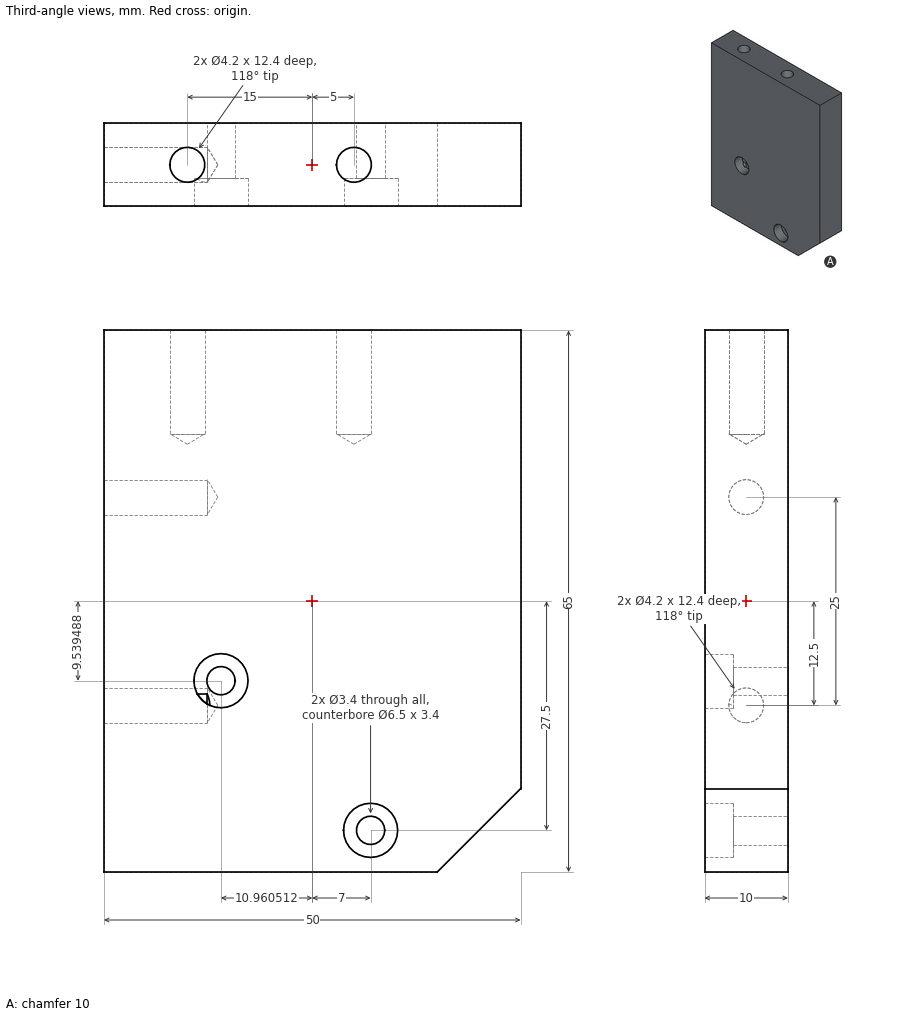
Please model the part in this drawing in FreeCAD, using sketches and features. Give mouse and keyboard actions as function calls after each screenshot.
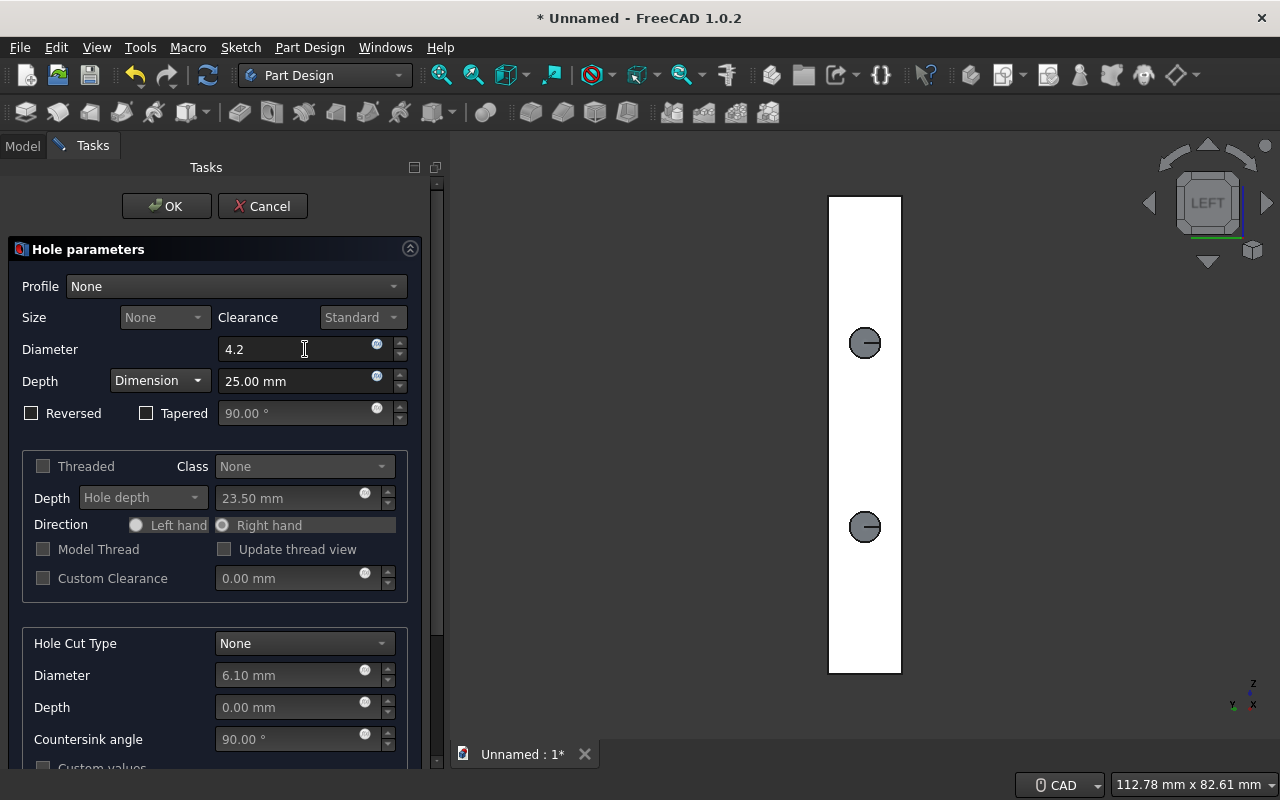
triple_click(305, 381)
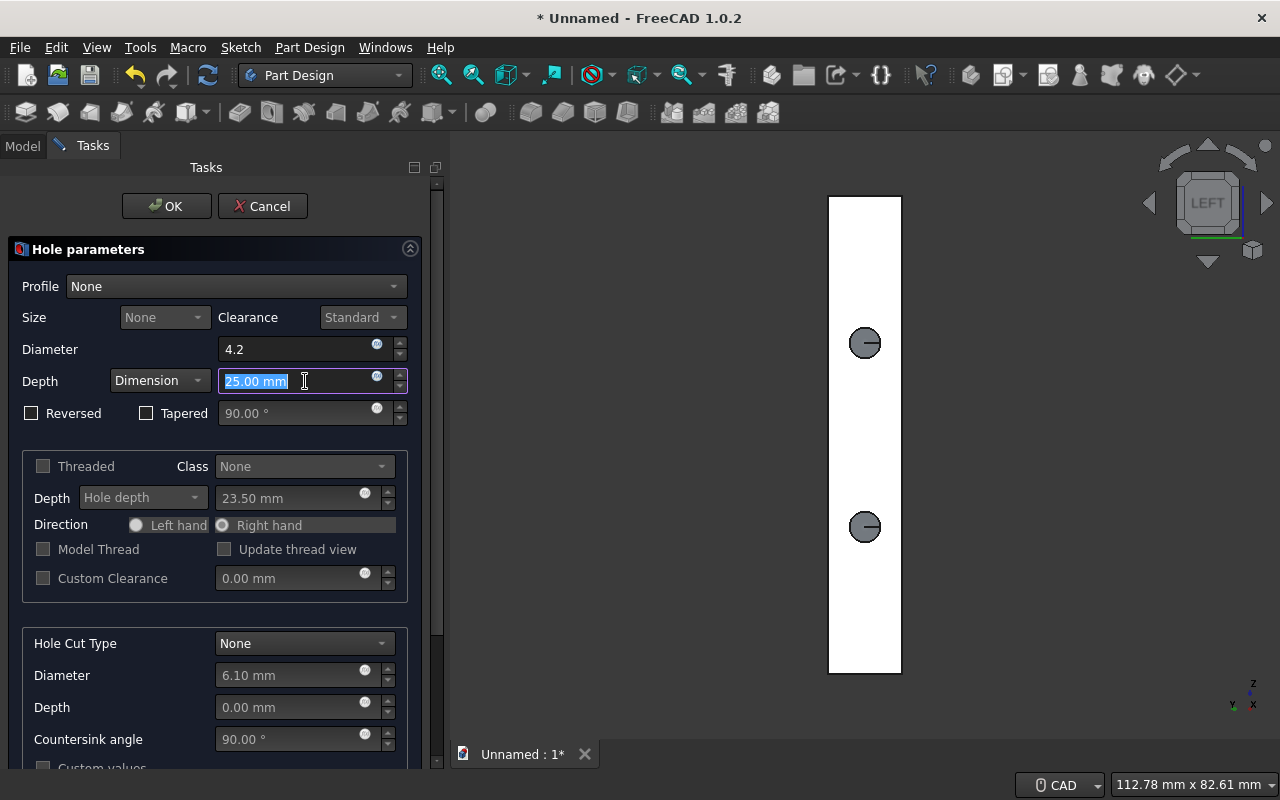
text(12.4)
key(Tab)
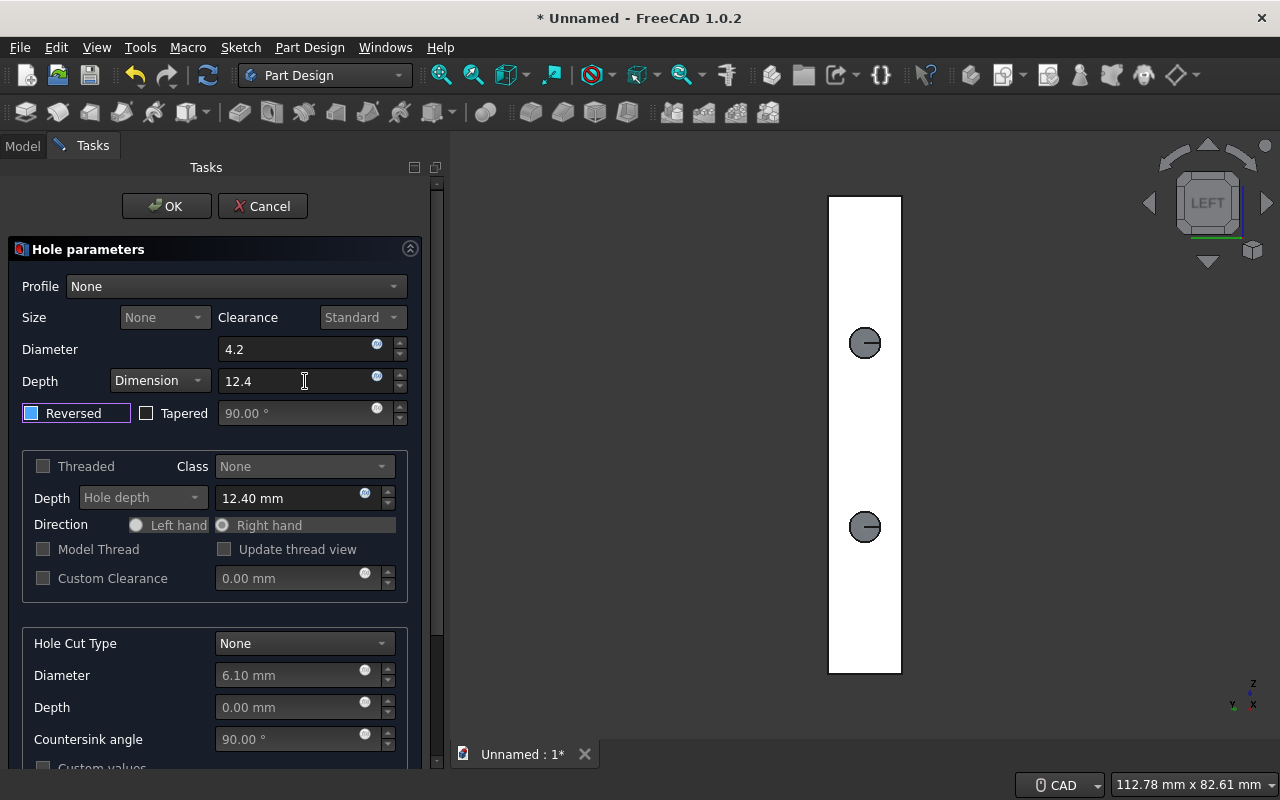
click(167, 206)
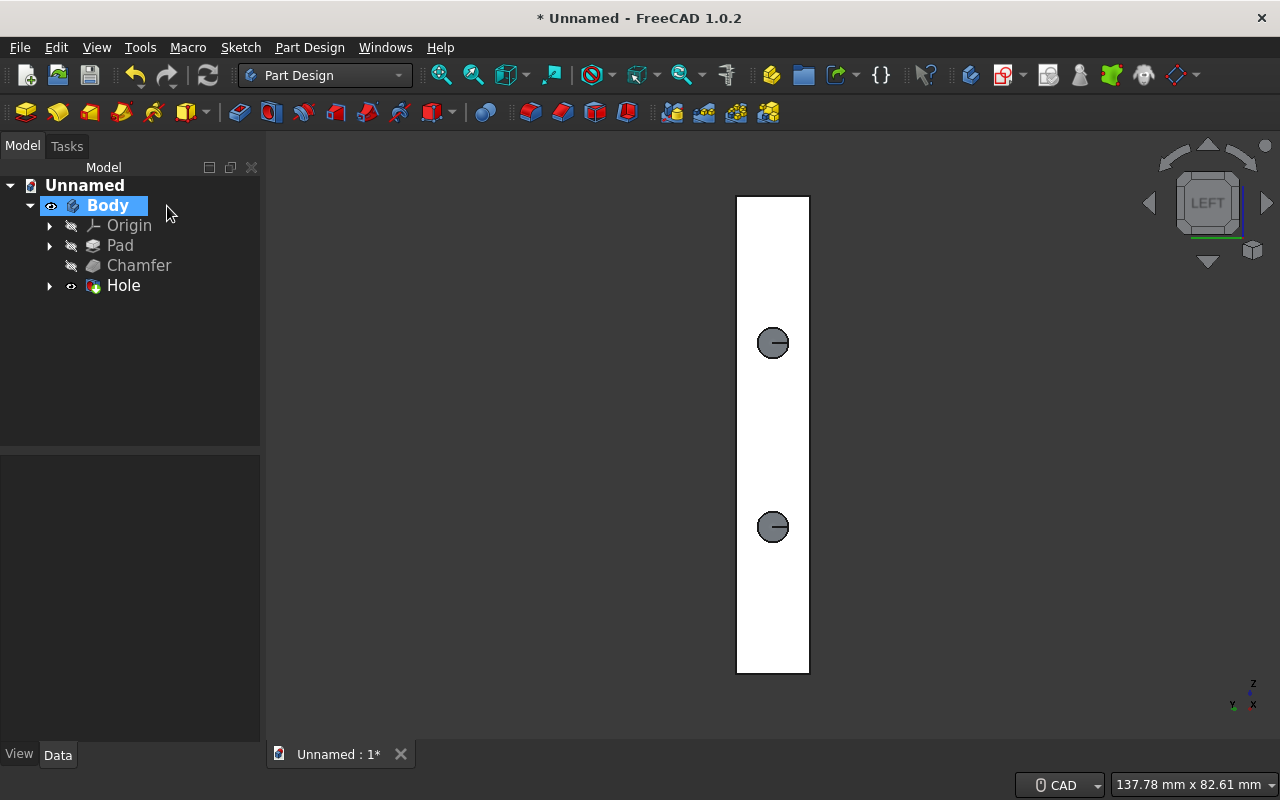
key(0)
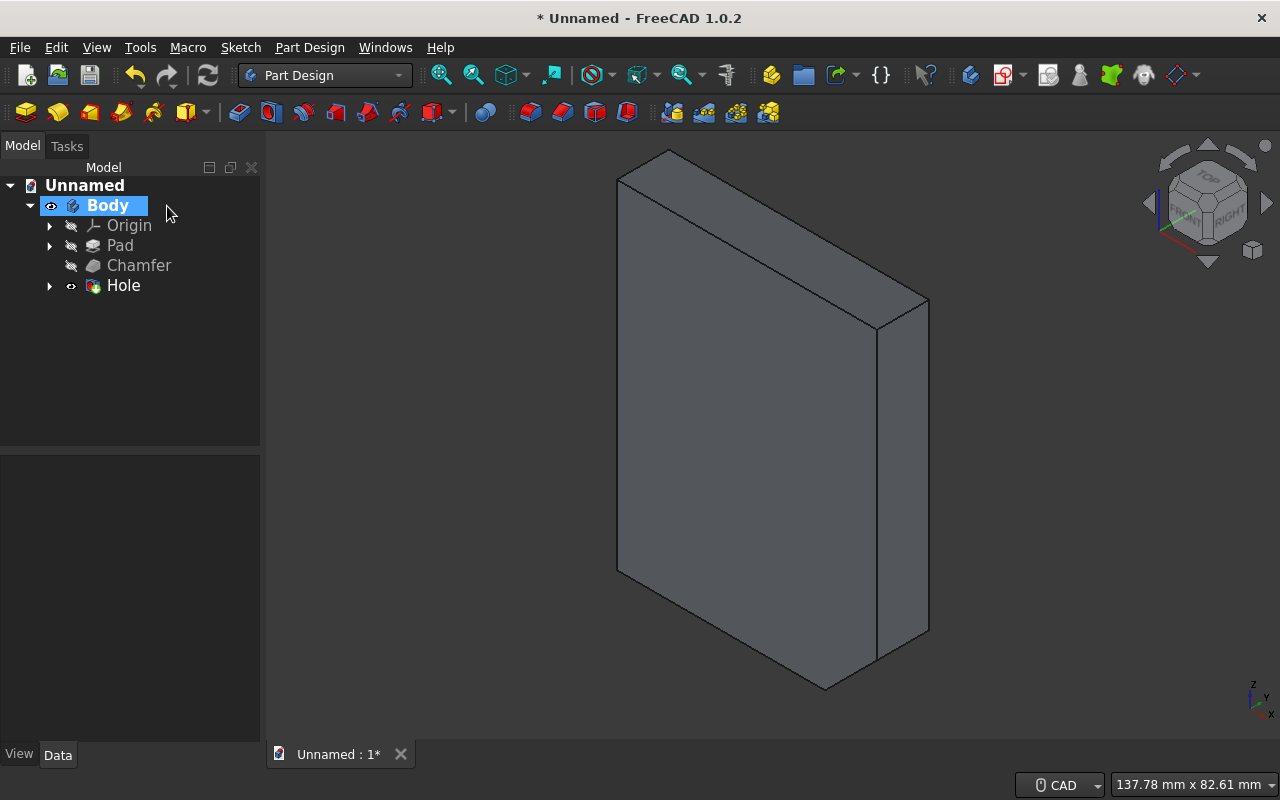
click(747, 449)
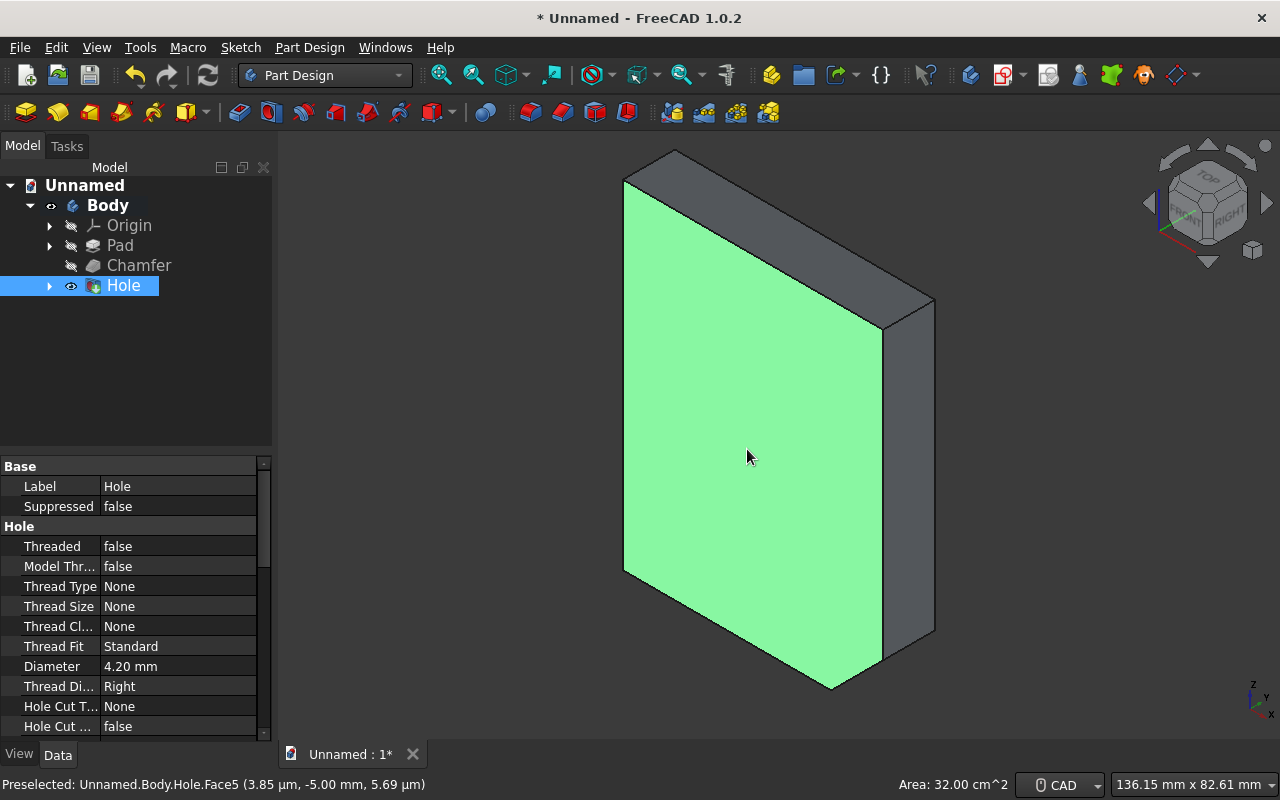
click(1004, 76)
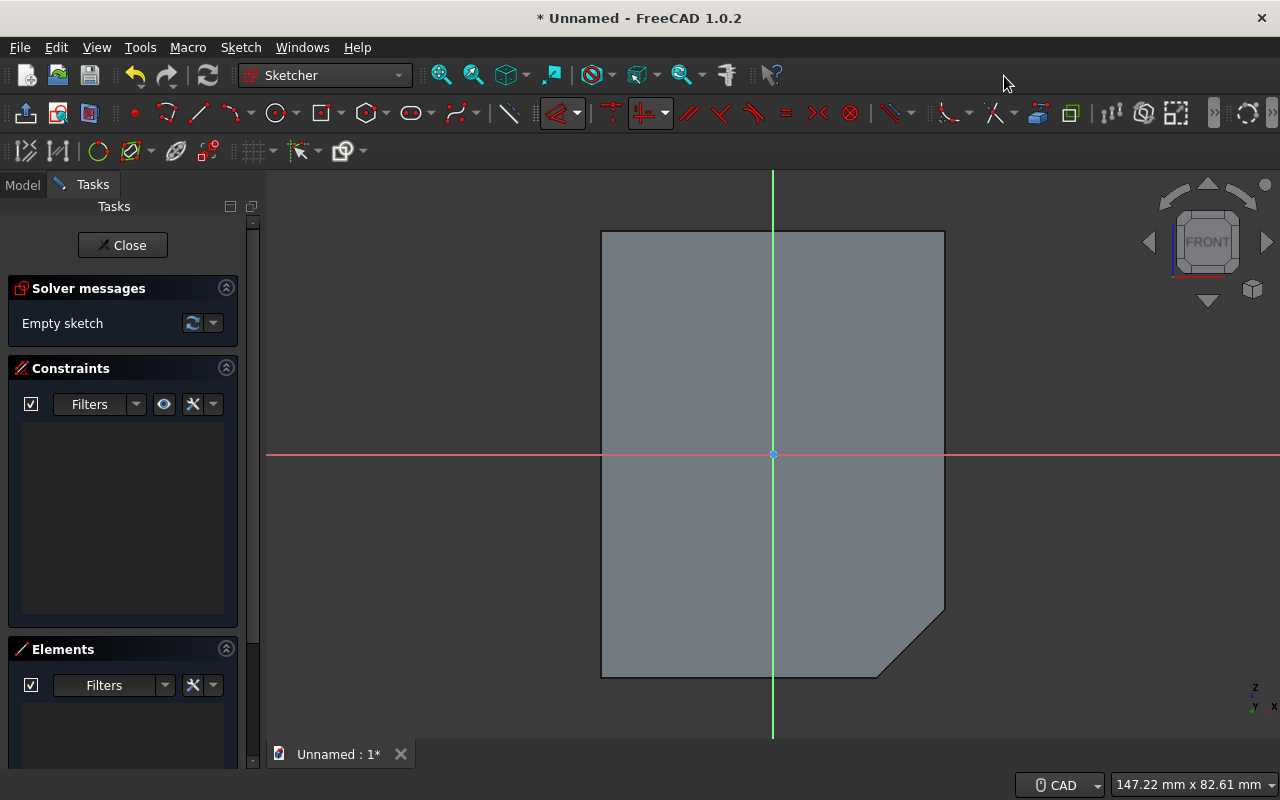
scroll(826, 677, up, 3)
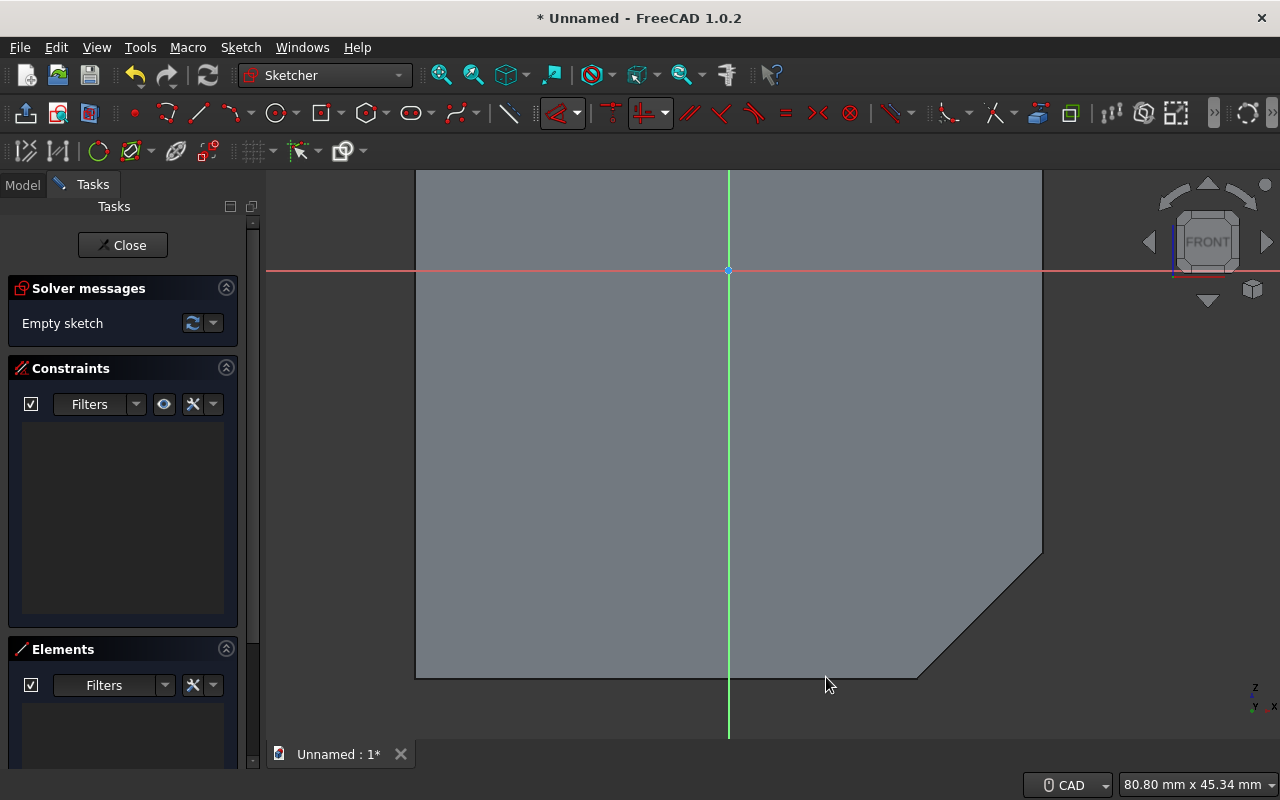
key(g)
key(c)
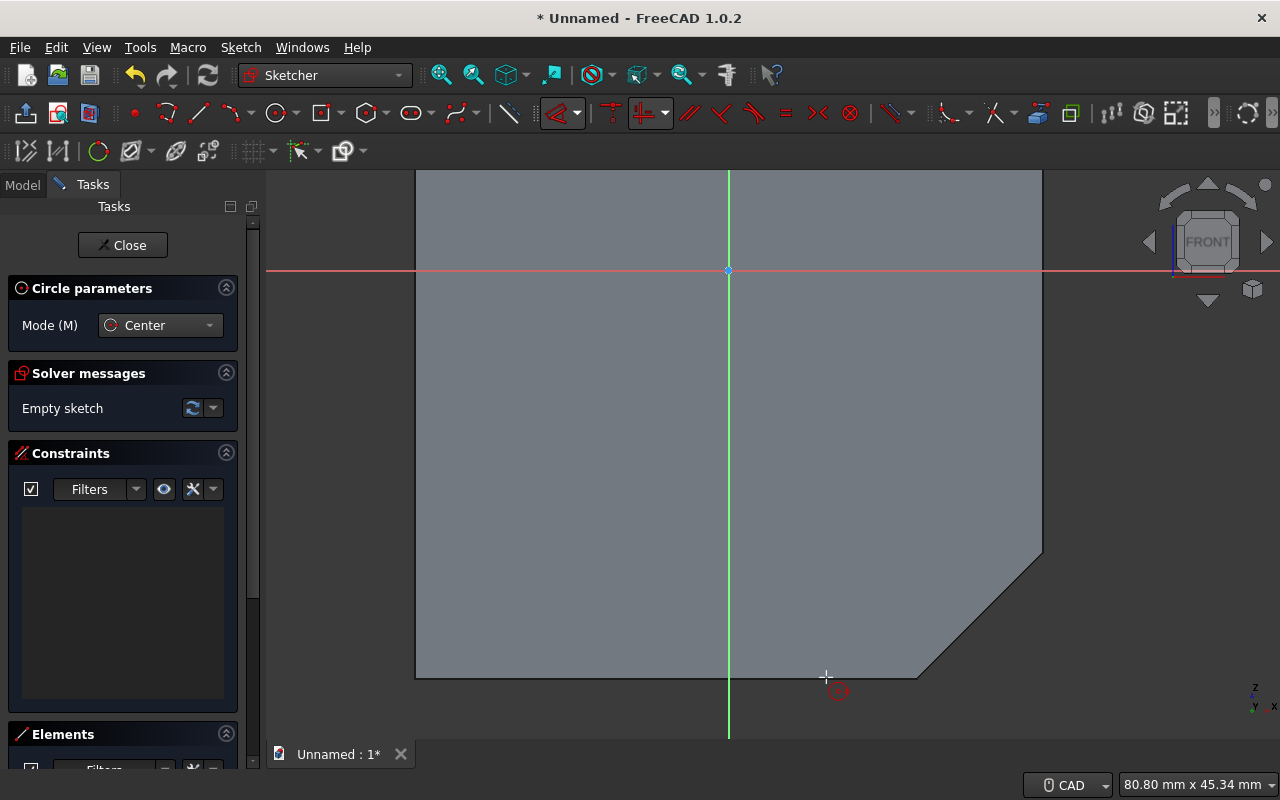
click(817, 616)
move(832, 601)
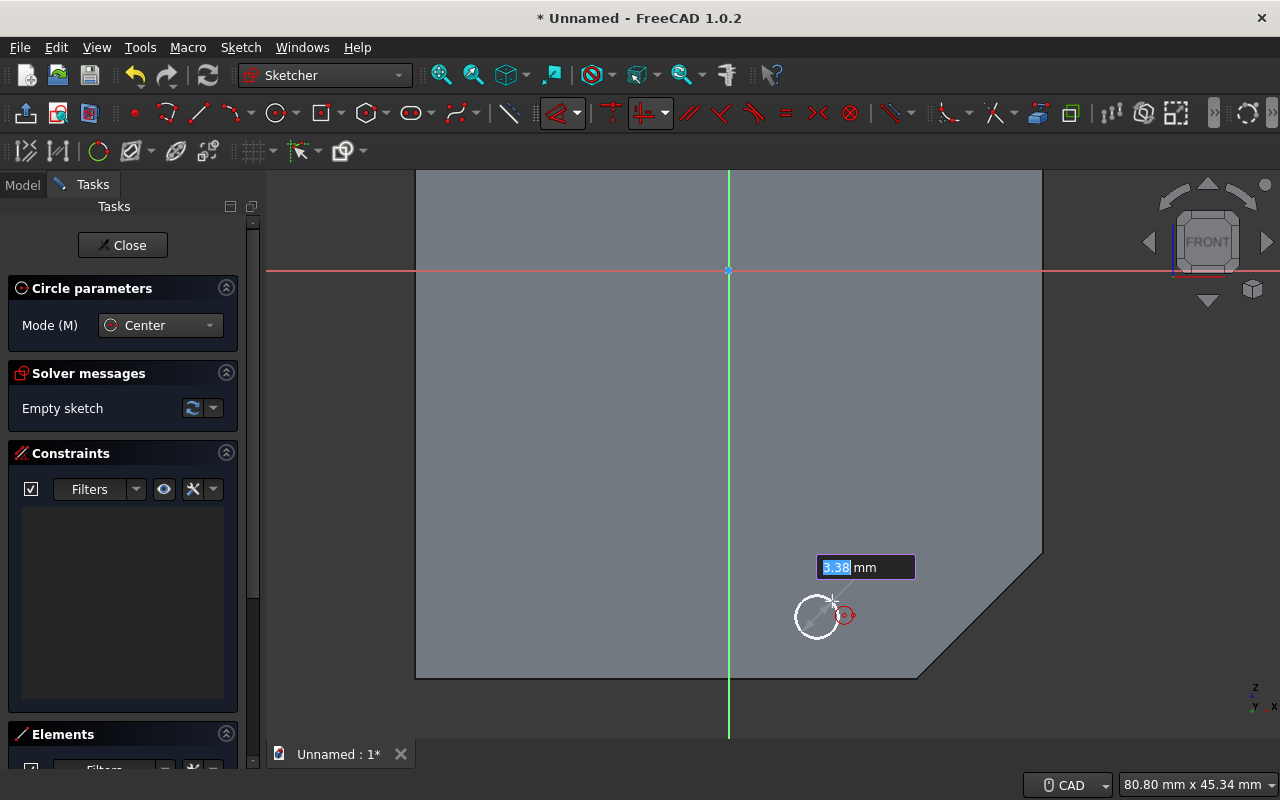
text(3.4)
key(Return)